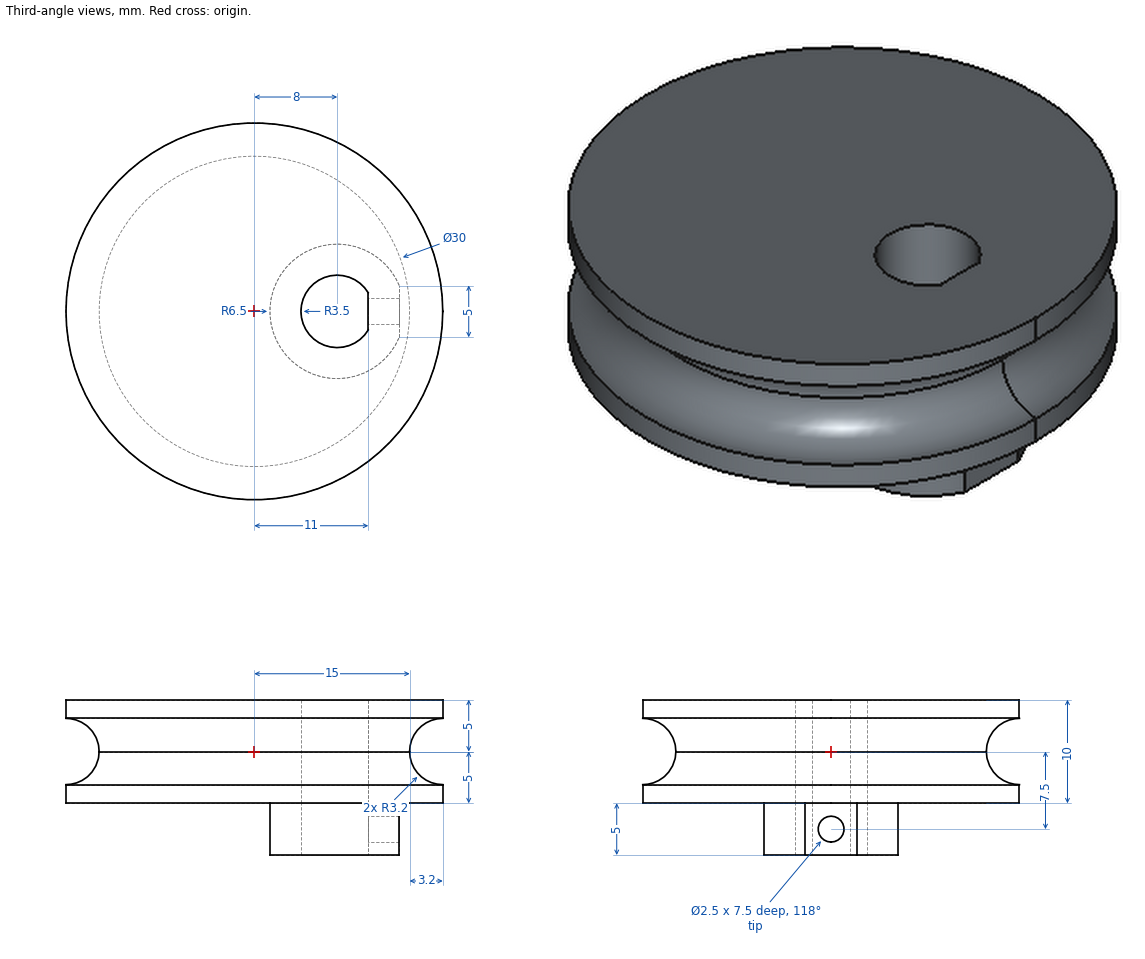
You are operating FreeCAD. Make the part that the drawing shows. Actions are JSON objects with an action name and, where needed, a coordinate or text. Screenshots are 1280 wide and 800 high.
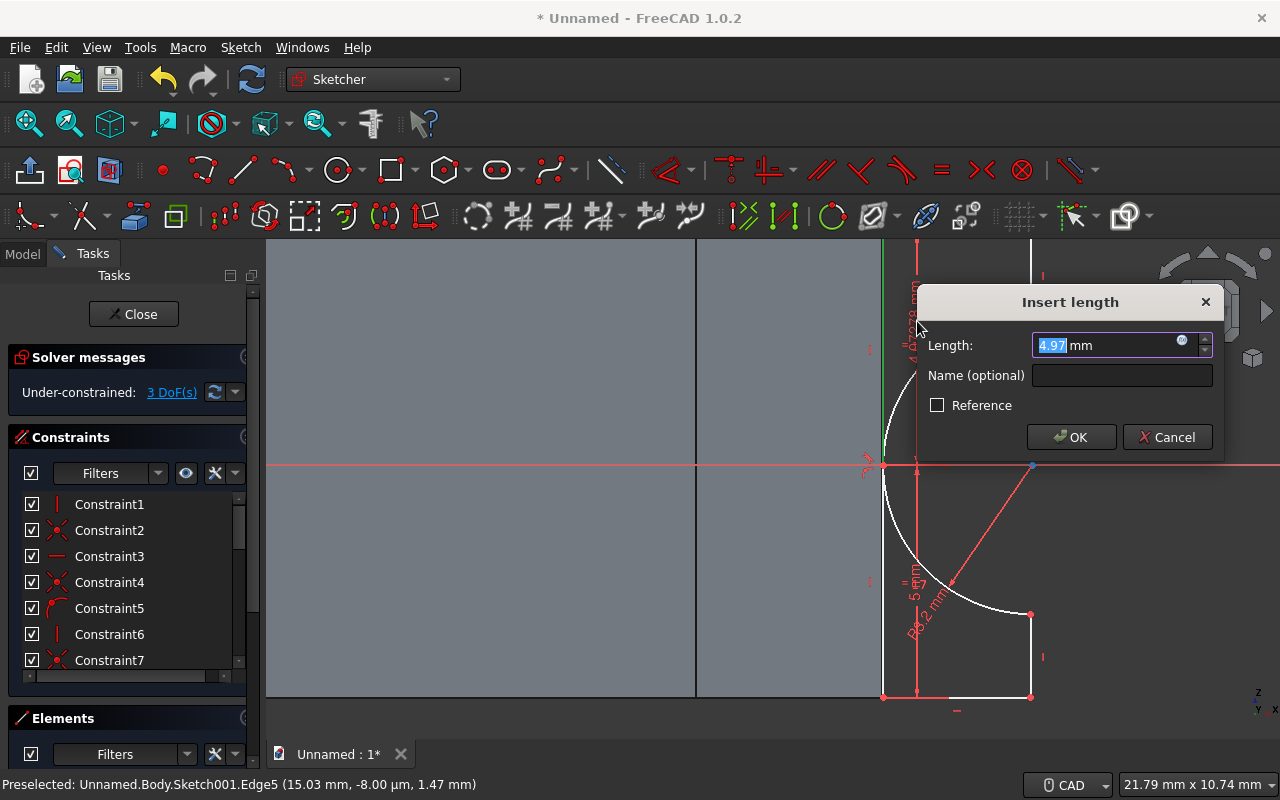
{"action": "type", "text": "5"}
{"action": "key", "text": "Return"}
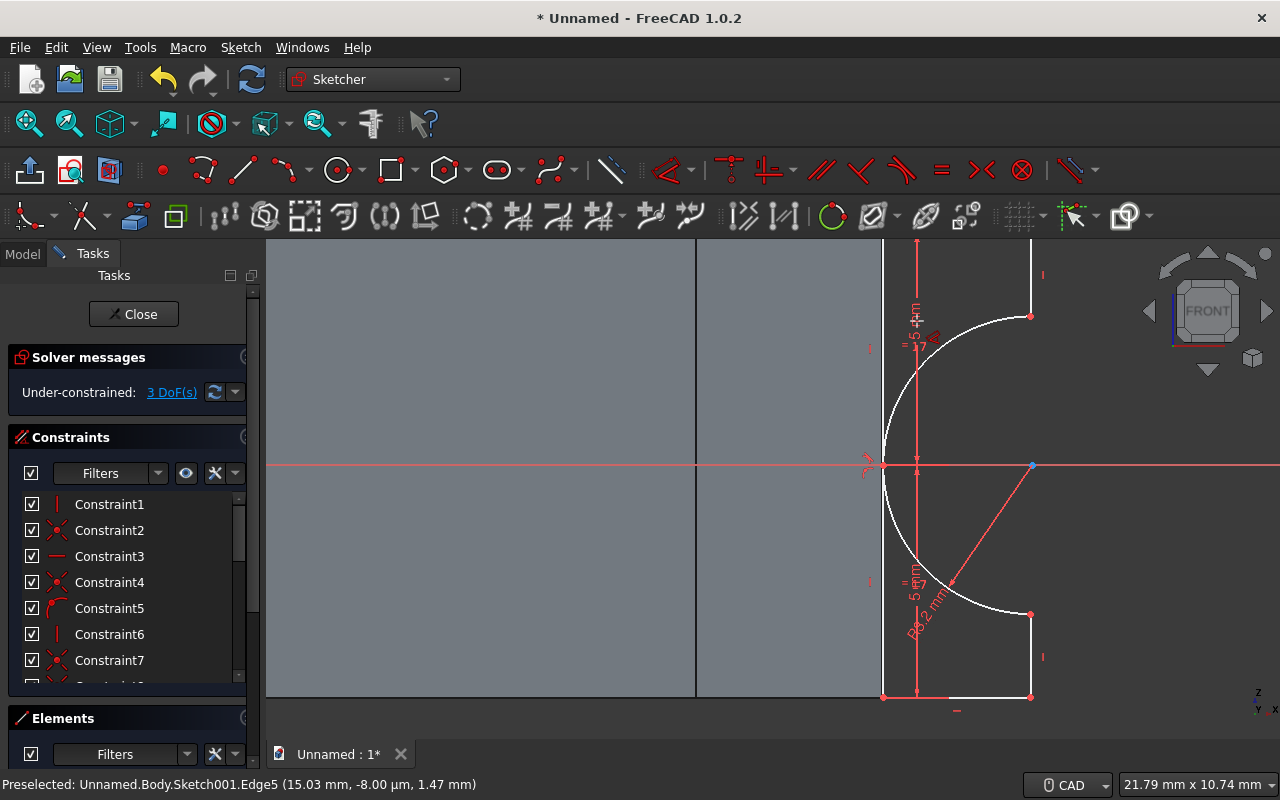
{"action": "left_click", "coordinate": [987, 698]}
{"action": "left_click", "coordinate": [957, 664]}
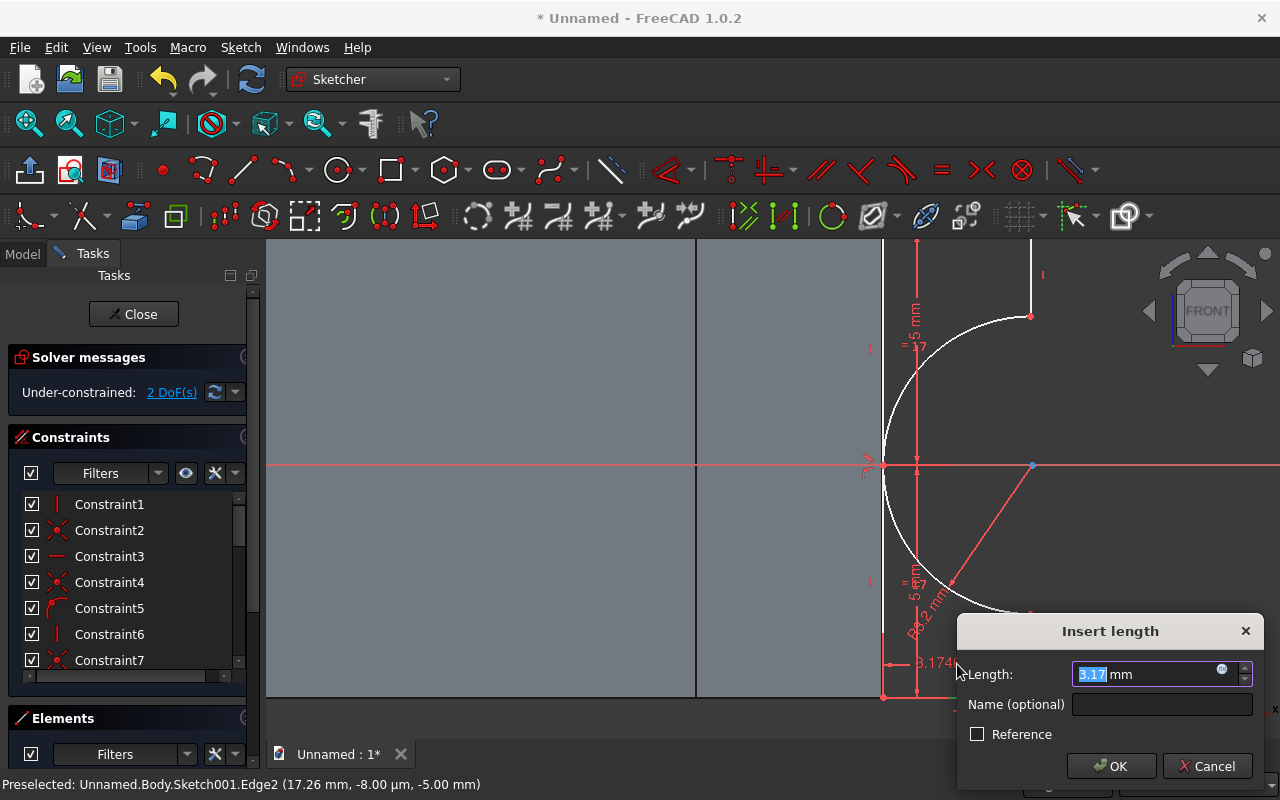
{"action": "type", "text": "3.2"}
{"action": "key", "text": "Return"}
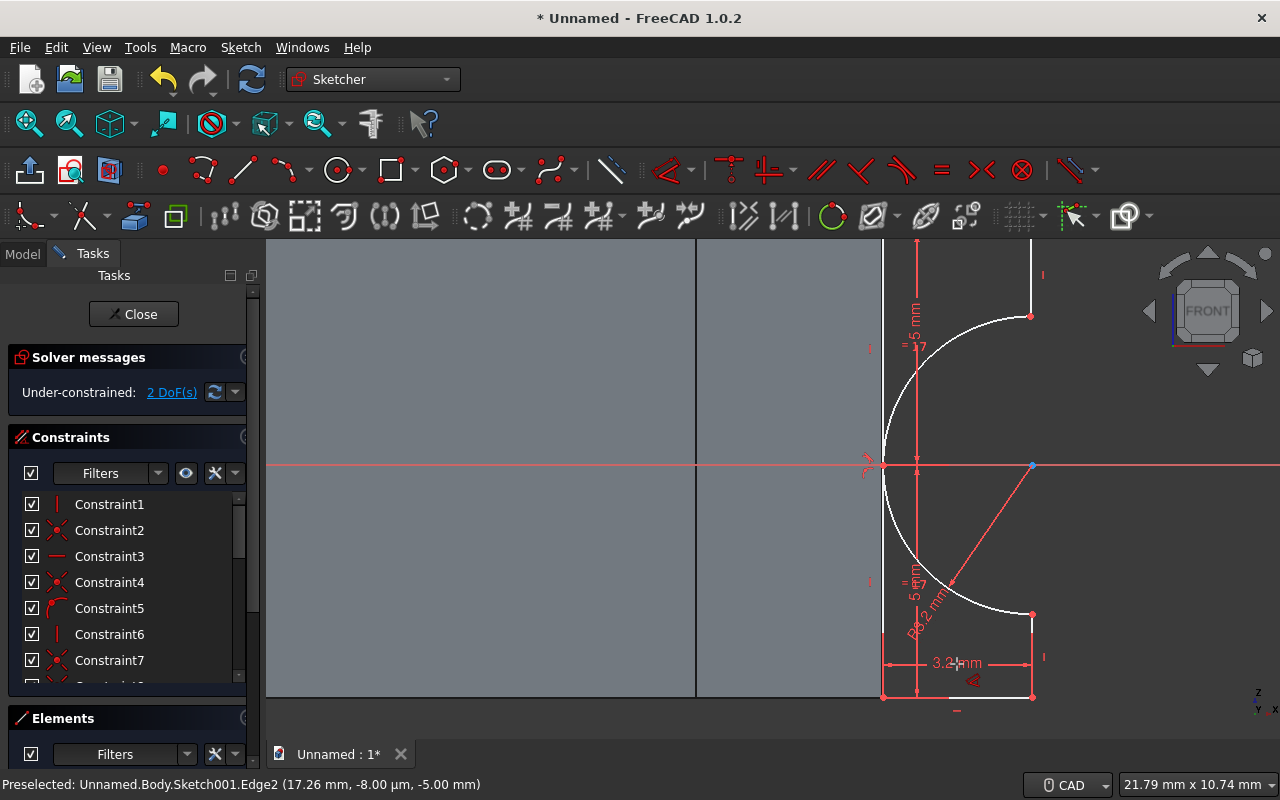
{"action": "scroll", "coordinate": [902, 537], "scroll_direction": "down", "scroll_amount": 2}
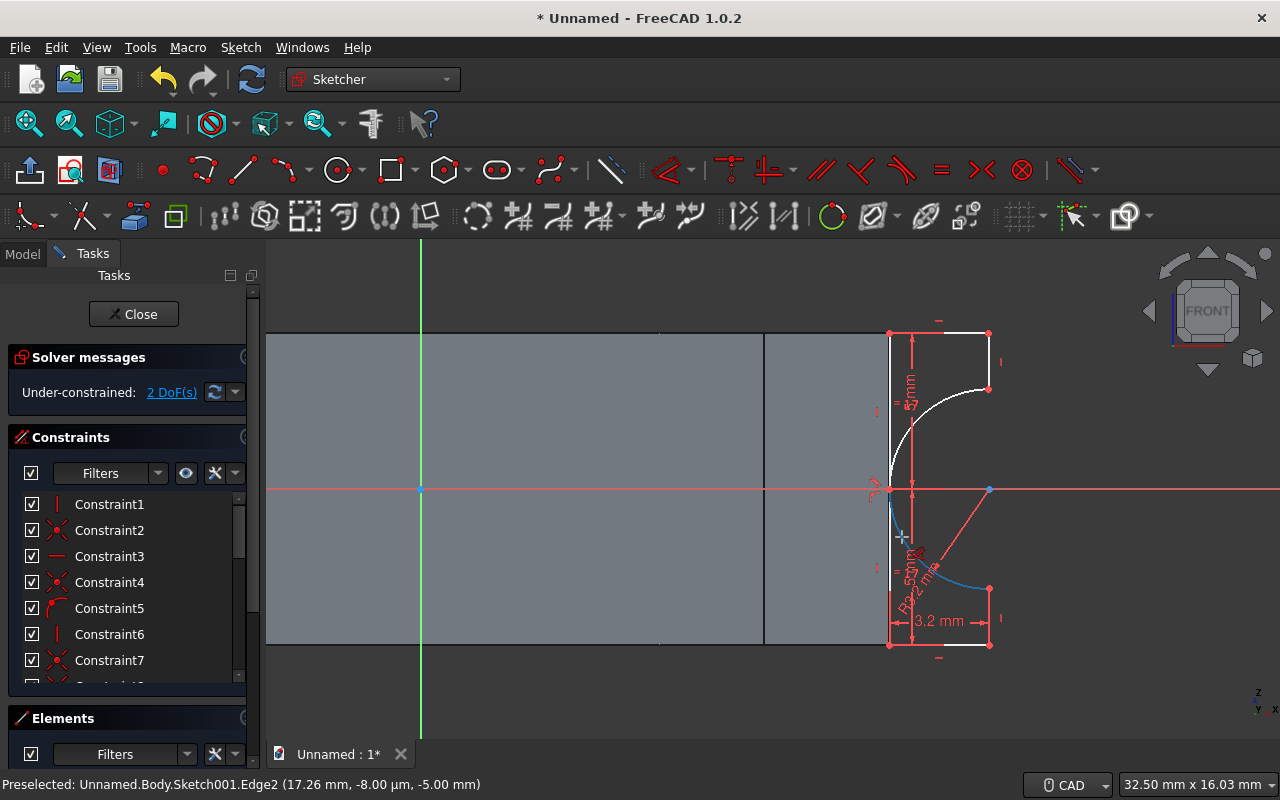
{"action": "left_click", "coordinate": [919, 333]}
{"action": "left_click", "coordinate": [939, 299]}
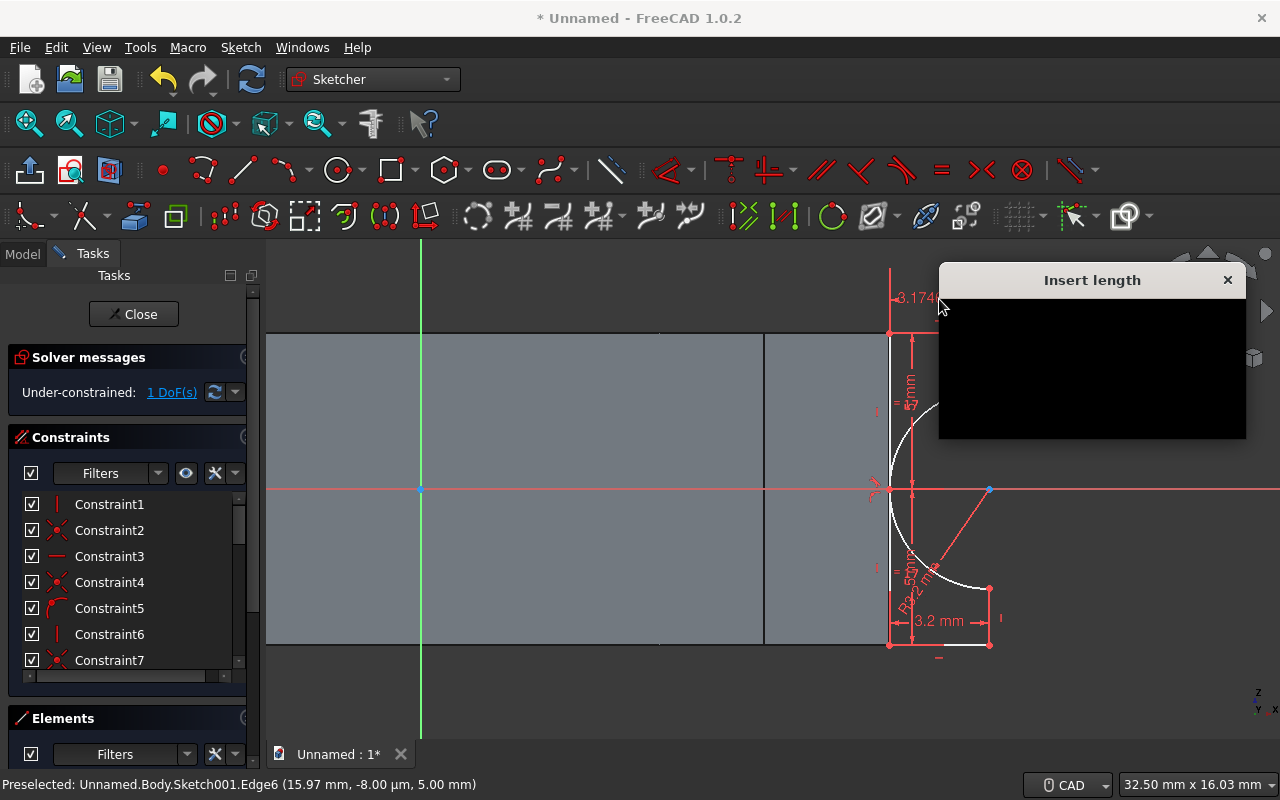
{"action": "type", "text": "3.2"}
{"action": "key", "text": "Return"}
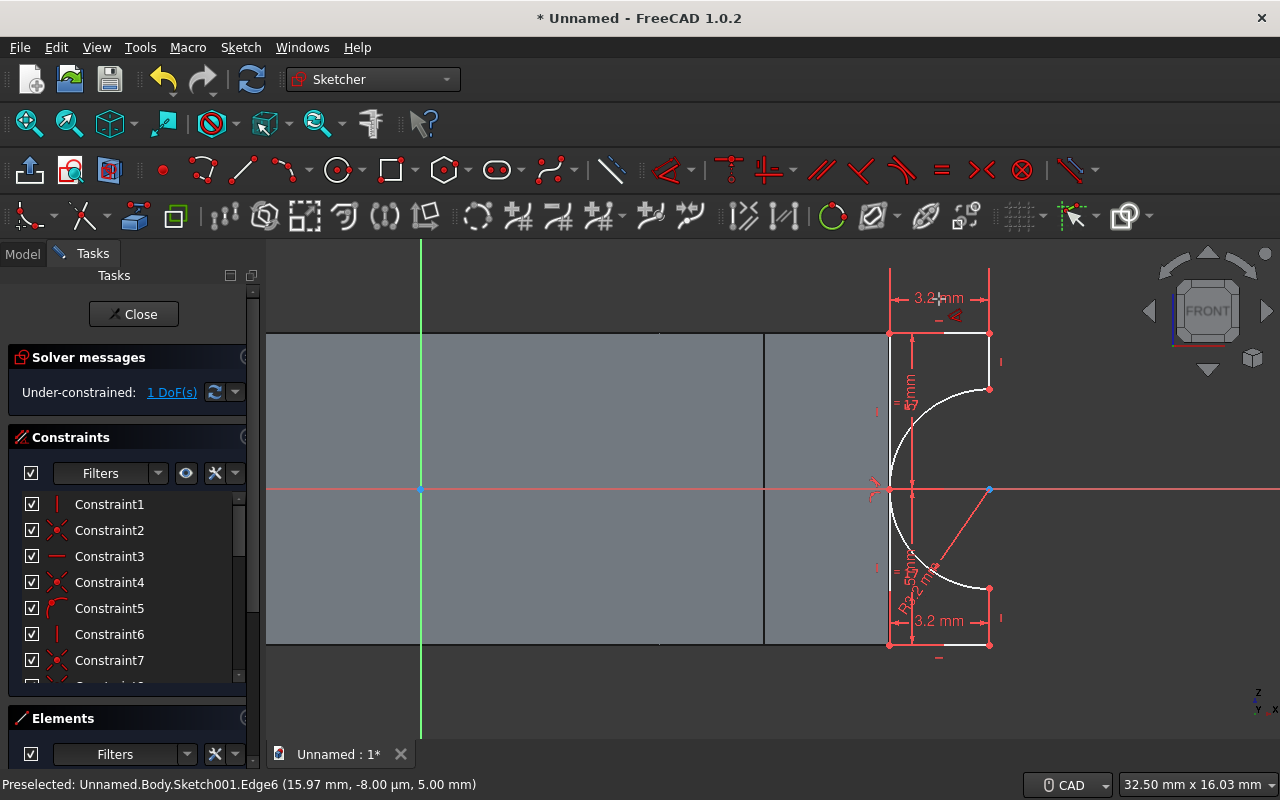
{"action": "left_click", "coordinate": [890, 645]}
{"action": "left_click", "coordinate": [655, 679]}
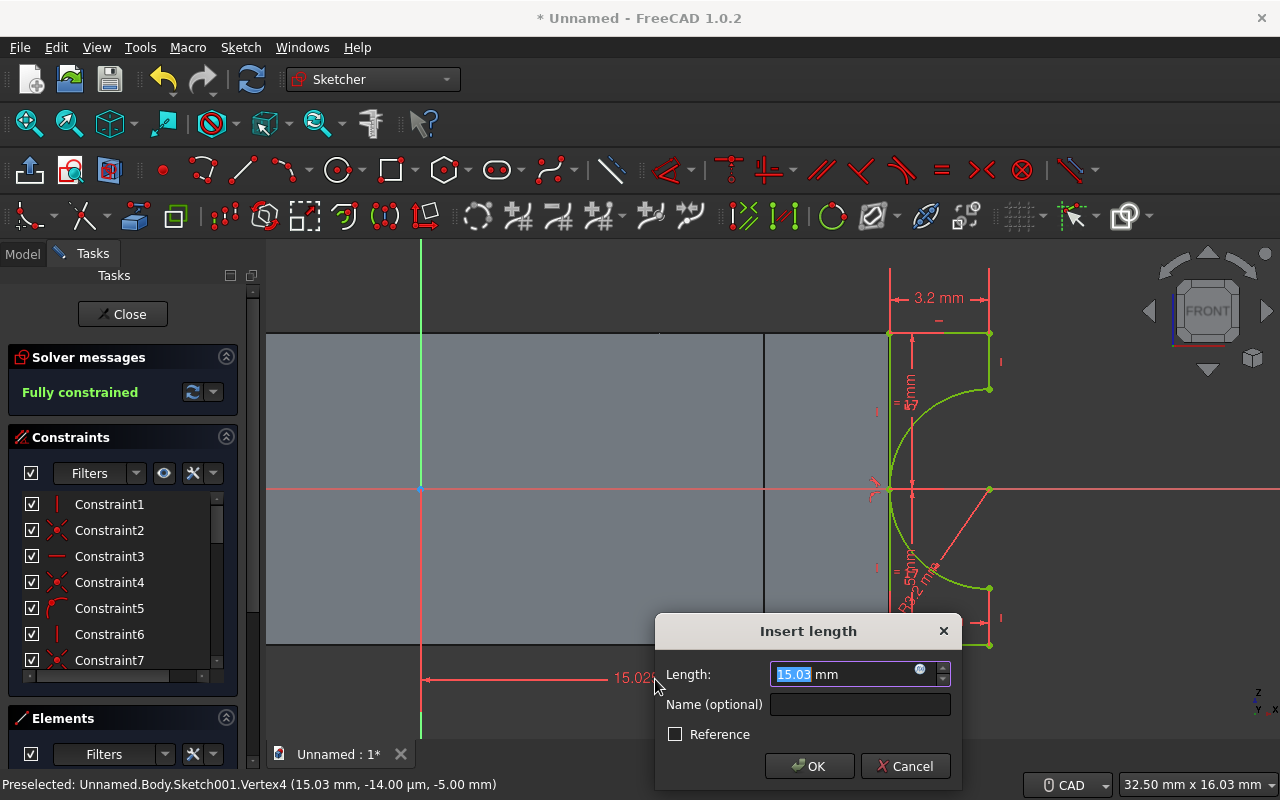
{"action": "type", "text": "15"}
{"action": "key", "text": "Return"}
{"action": "key", "text": "Escape"}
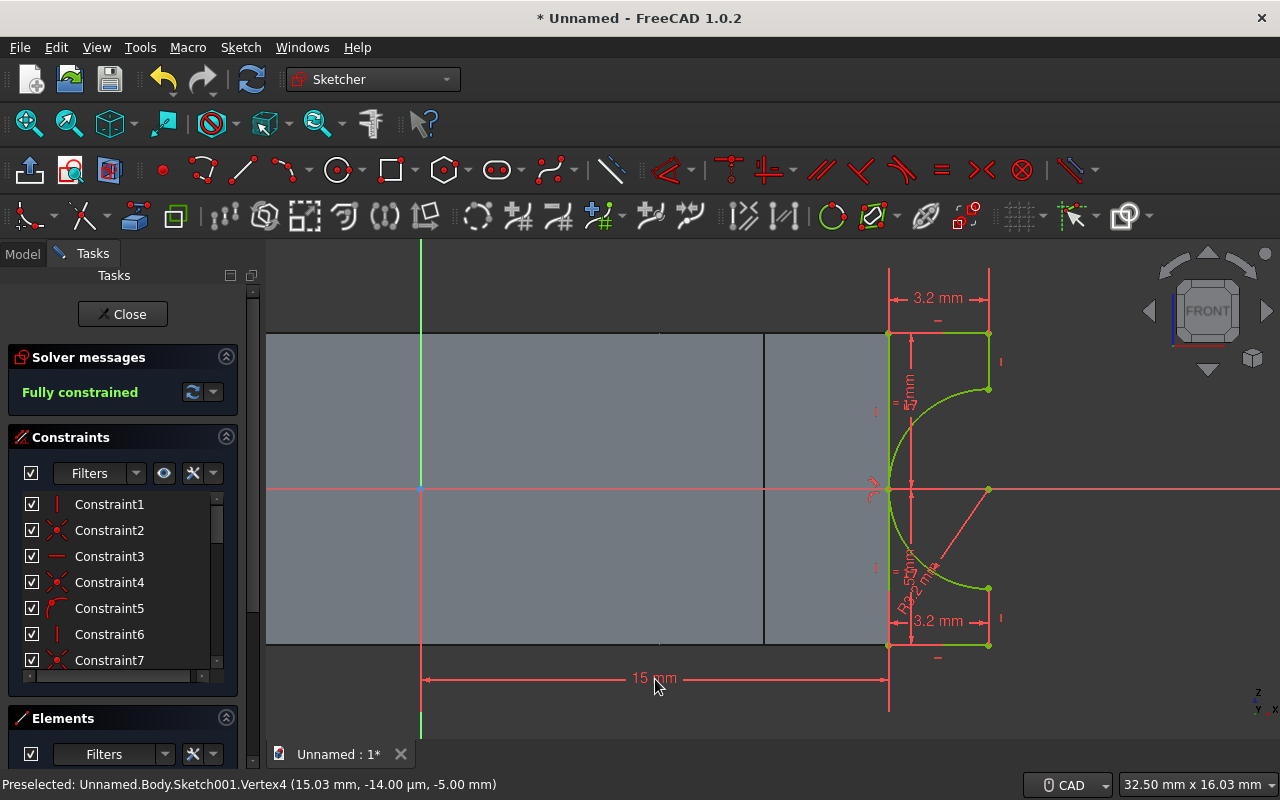
{"action": "left_click", "coordinate": [123, 314]}